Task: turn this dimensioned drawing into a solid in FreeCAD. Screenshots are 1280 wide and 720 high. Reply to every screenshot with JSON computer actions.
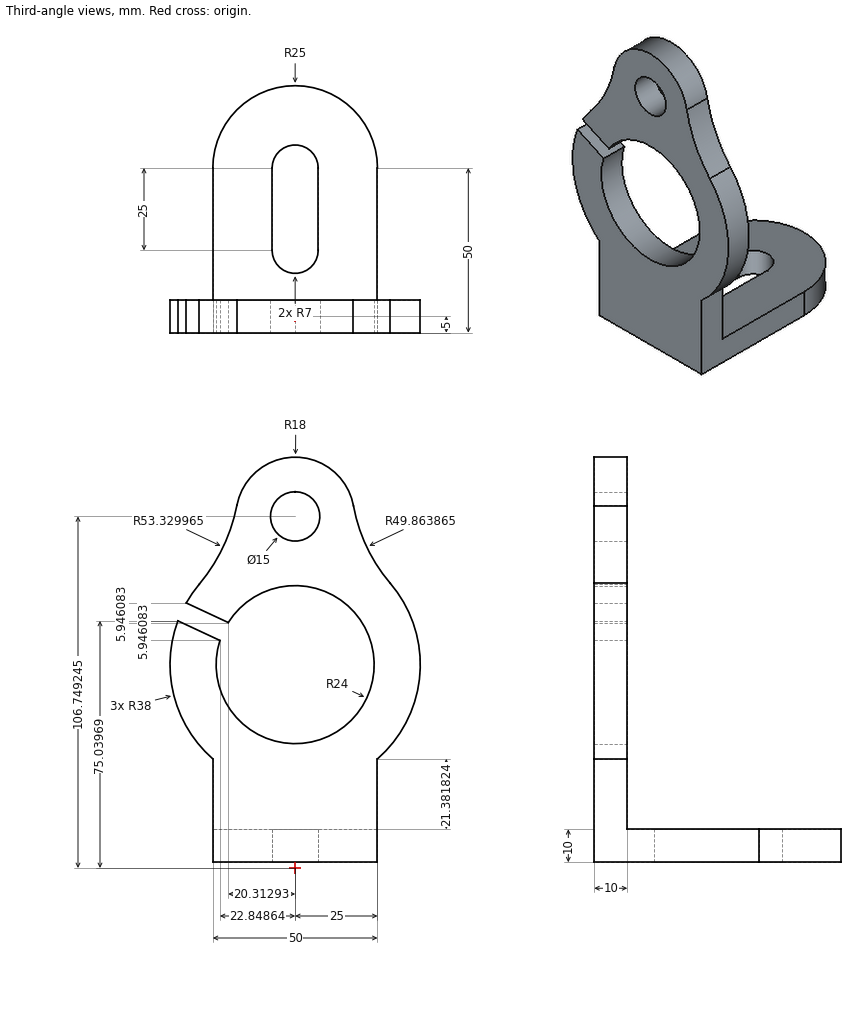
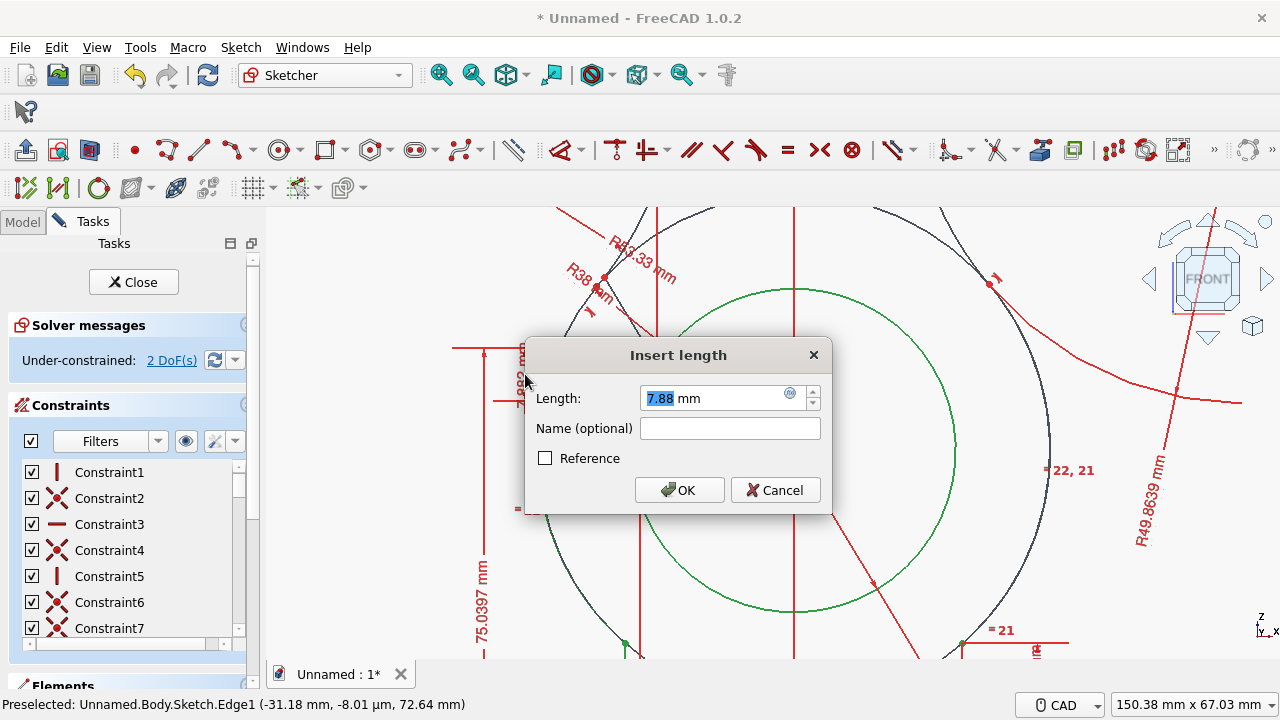
{"action": "type", "text": "5.946083"}
{"action": "key", "text": "Return"}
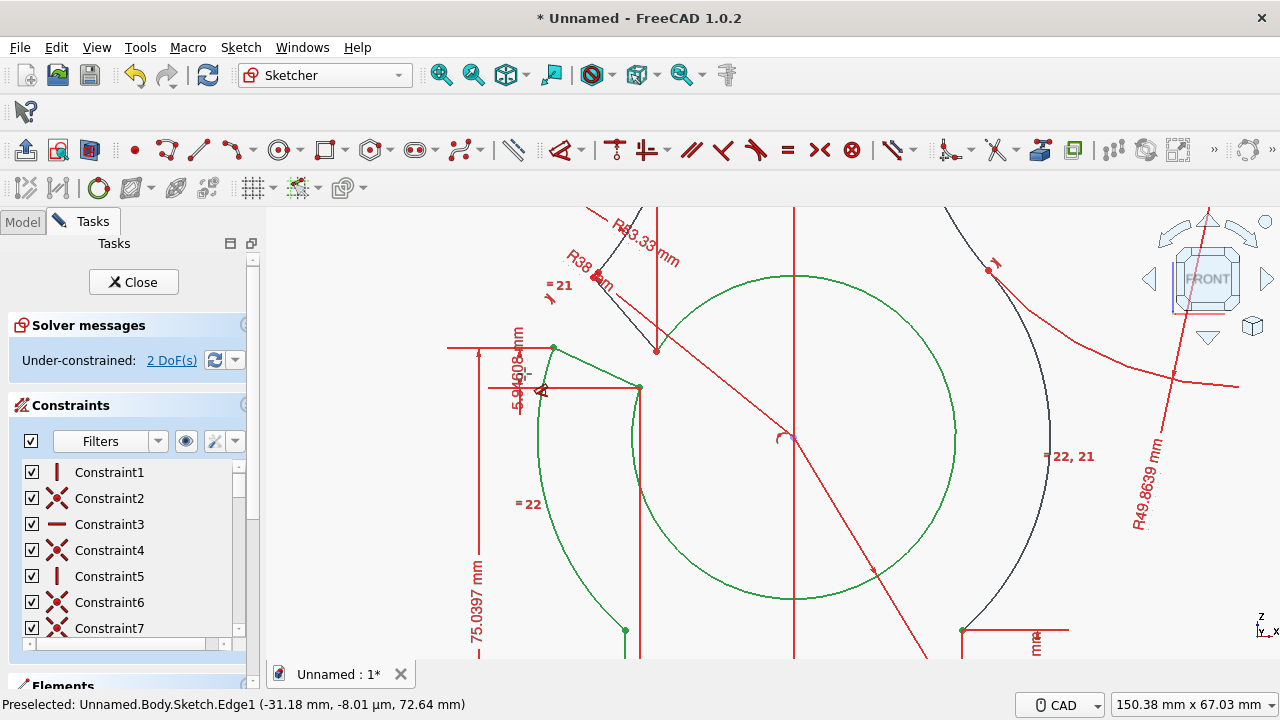
{"action": "left_click", "coordinate": [638, 329]}
{"action": "left_click", "coordinate": [560, 314]}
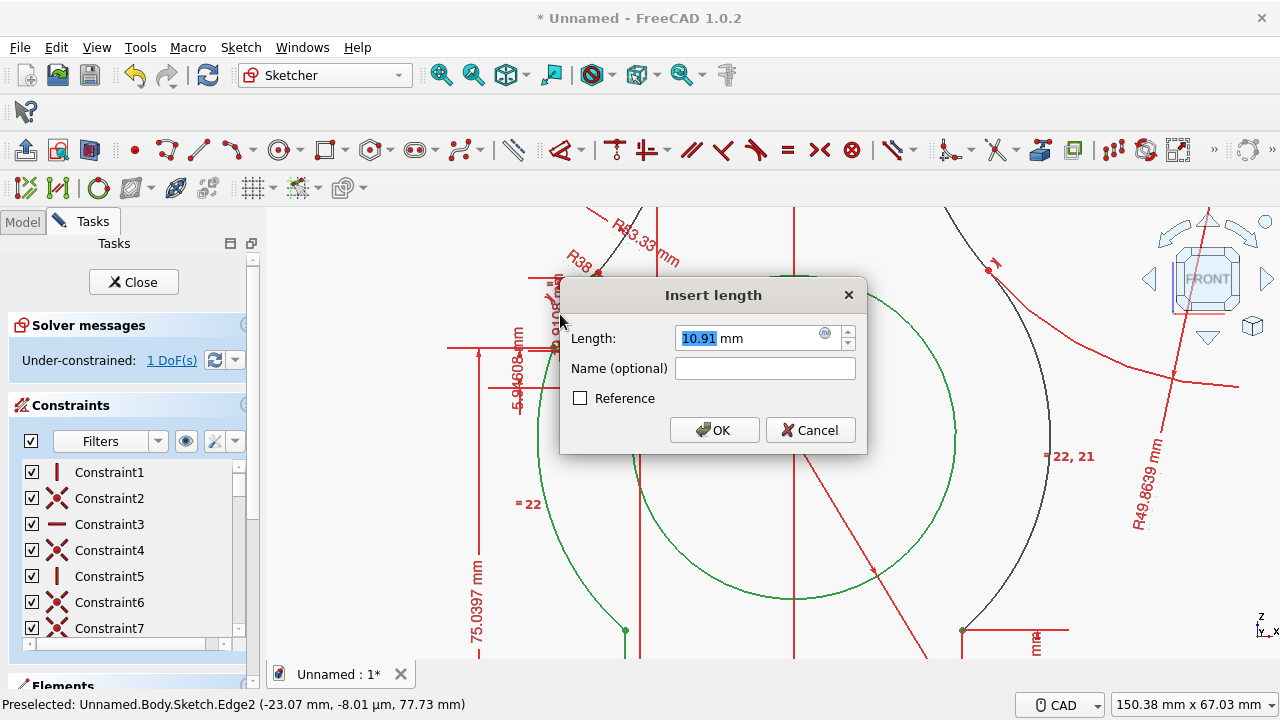
{"action": "type", "text": "5.946083"}
{"action": "key", "text": "Return"}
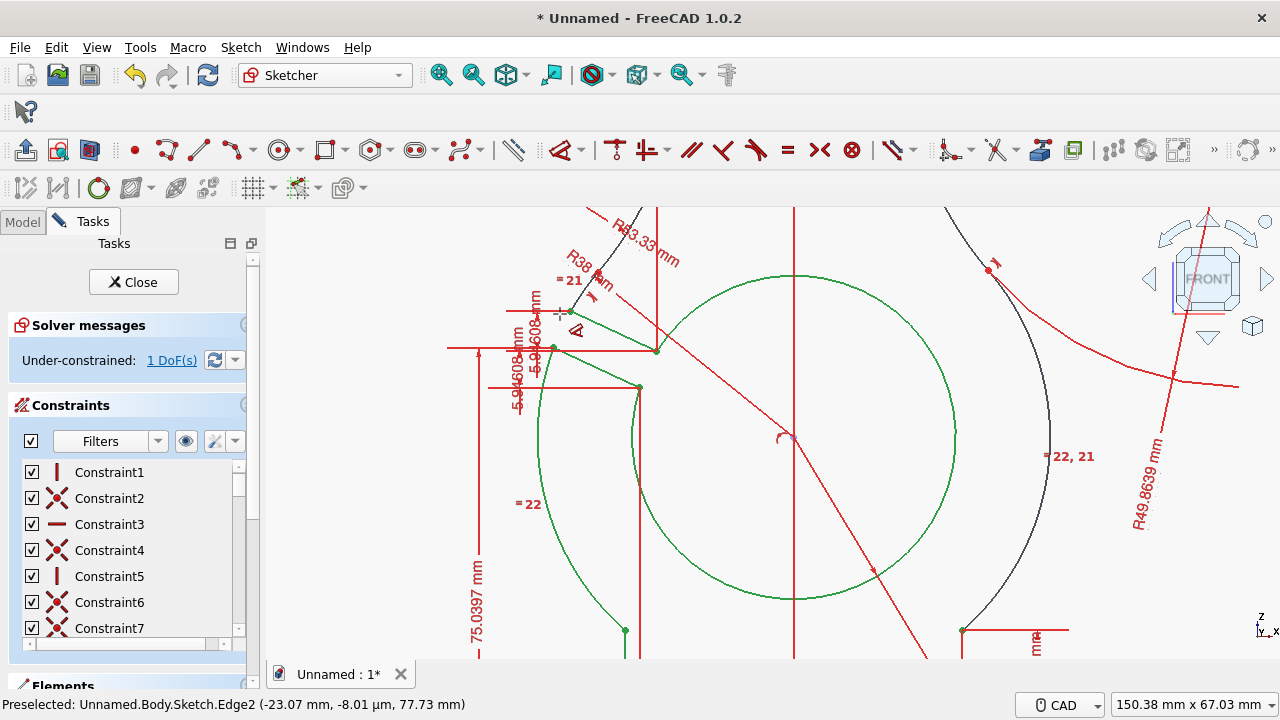
{"action": "scroll", "coordinate": [664, 433], "scroll_direction": "down", "scroll_amount": 6}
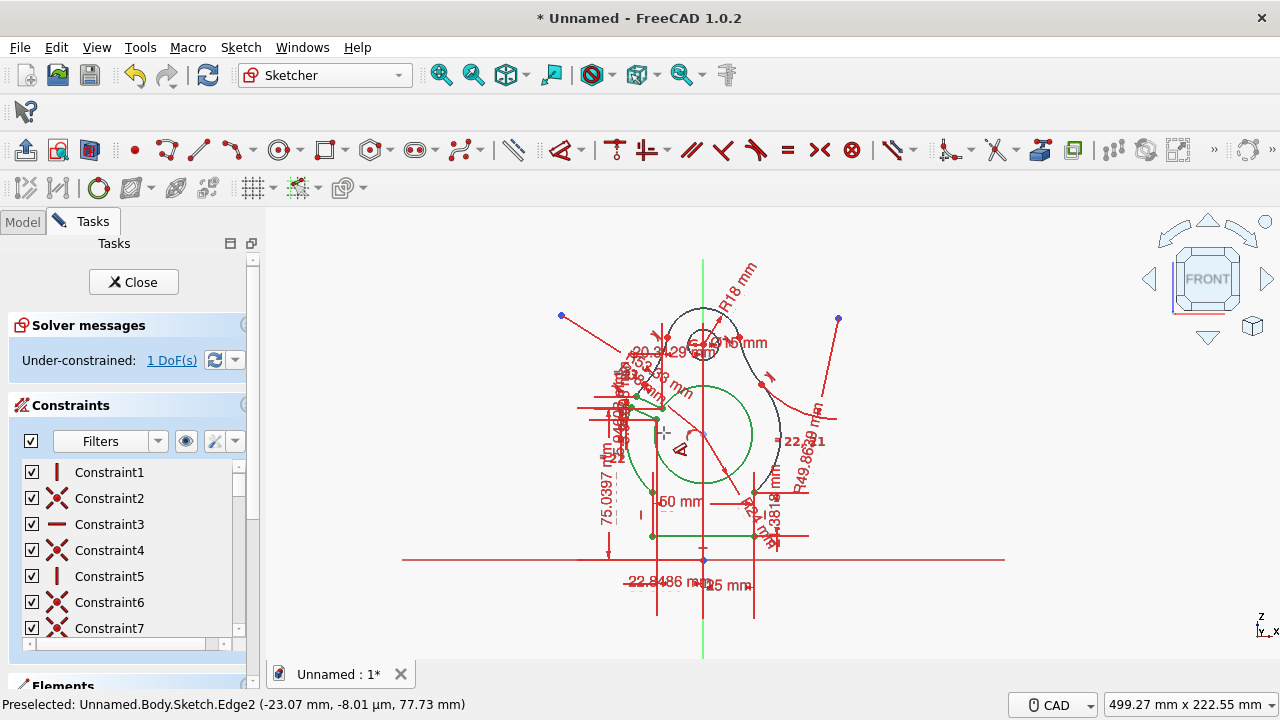
{"action": "left_click", "coordinate": [703, 345]}
{"action": "left_click", "coordinate": [737, 377]}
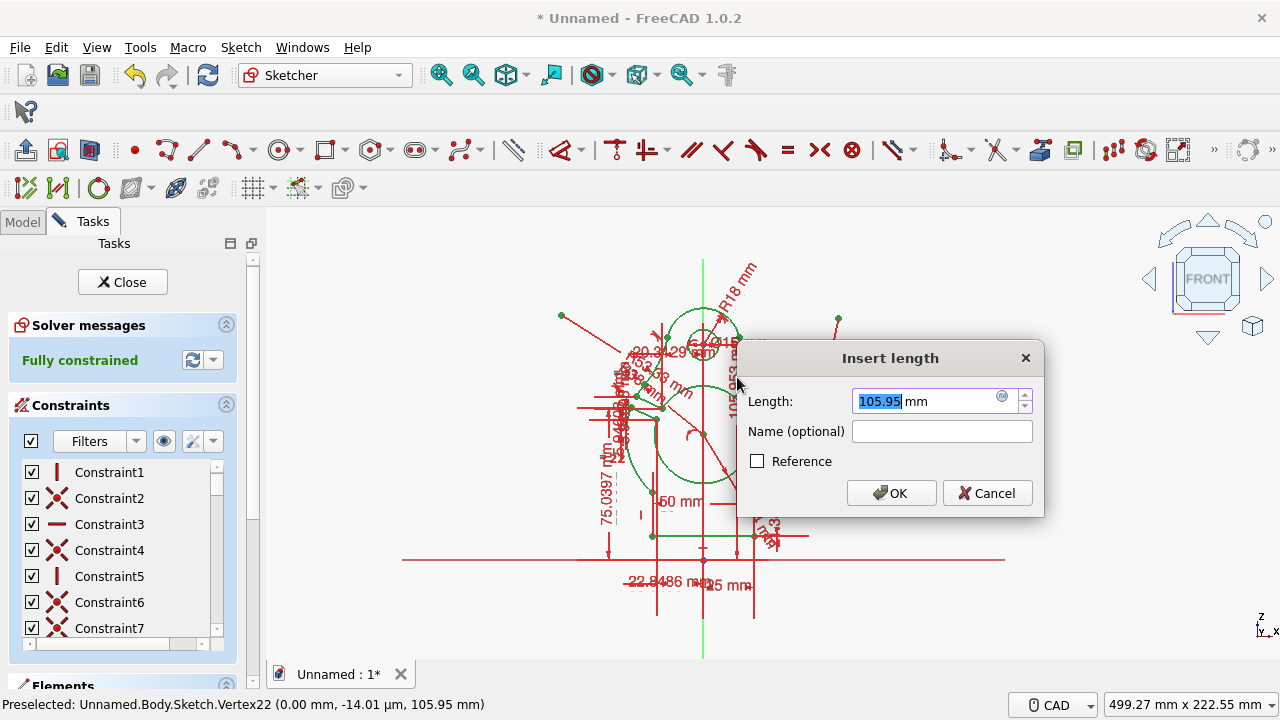
{"action": "type", "text": "106.749245"}
{"action": "key", "text": "Return"}
{"action": "key", "text": "Escape"}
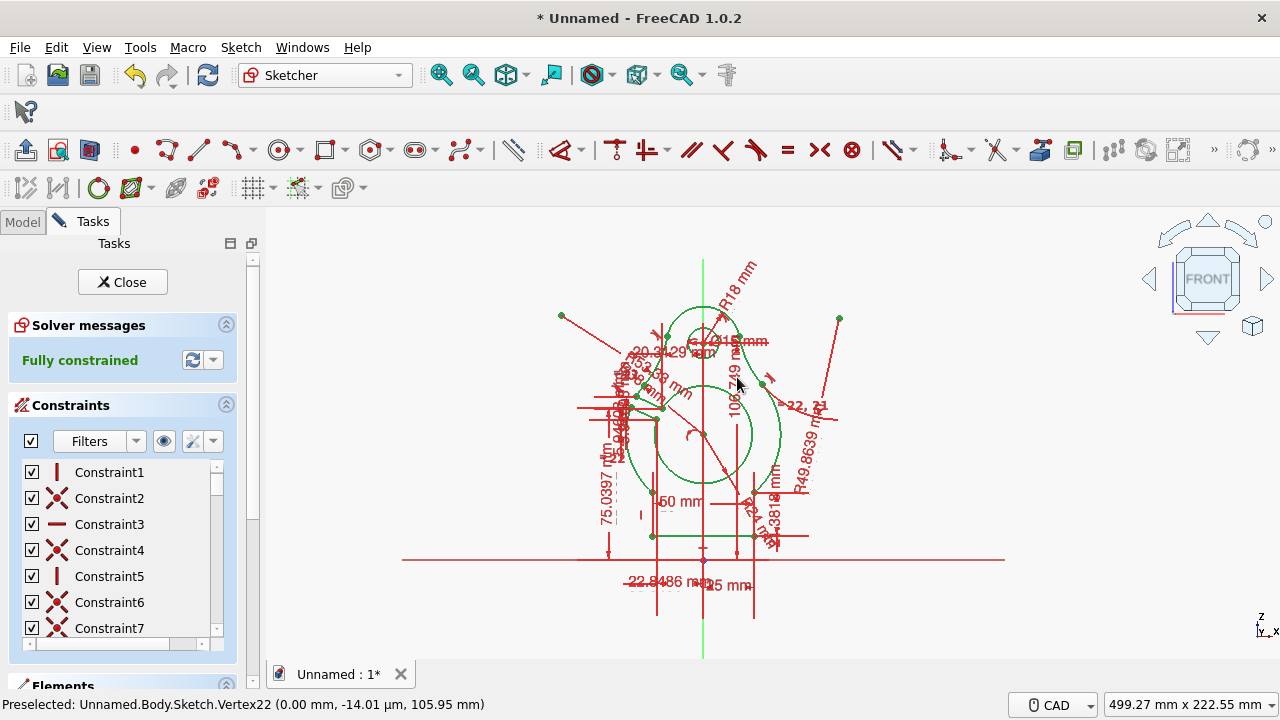
{"action": "left_click", "coordinate": [123, 282]}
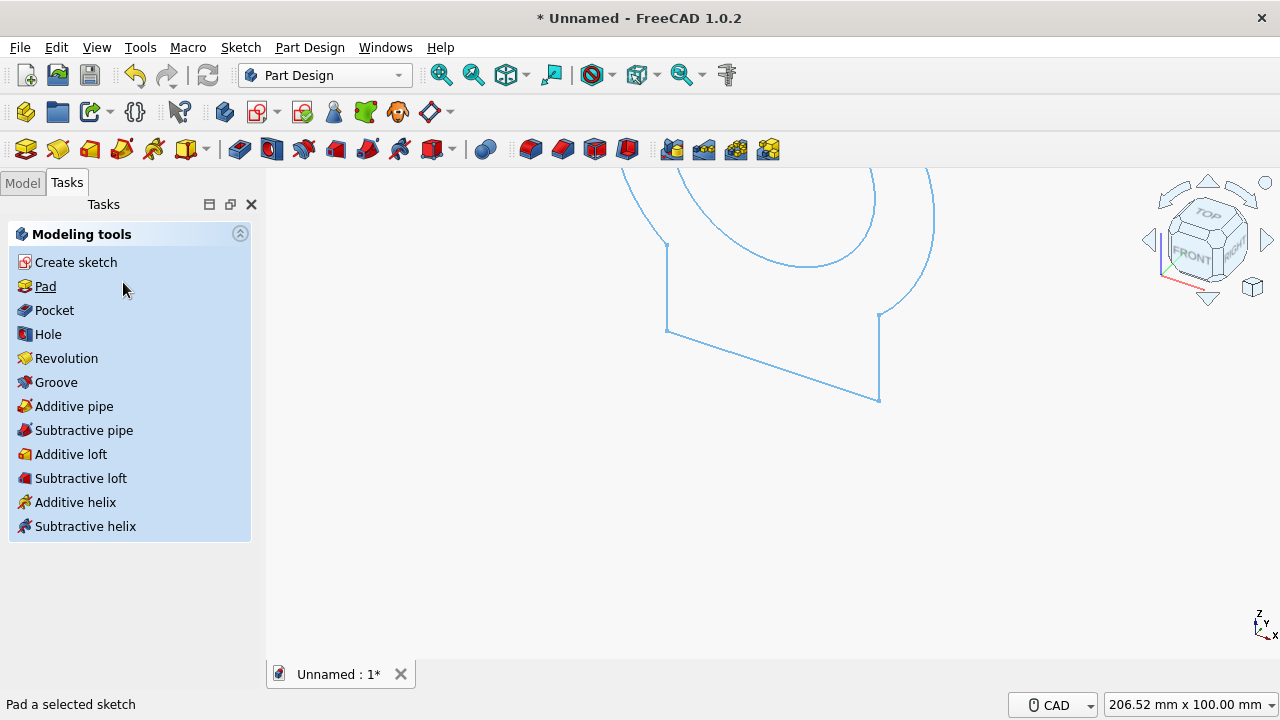
{"action": "left_click", "coordinate": [26, 150]}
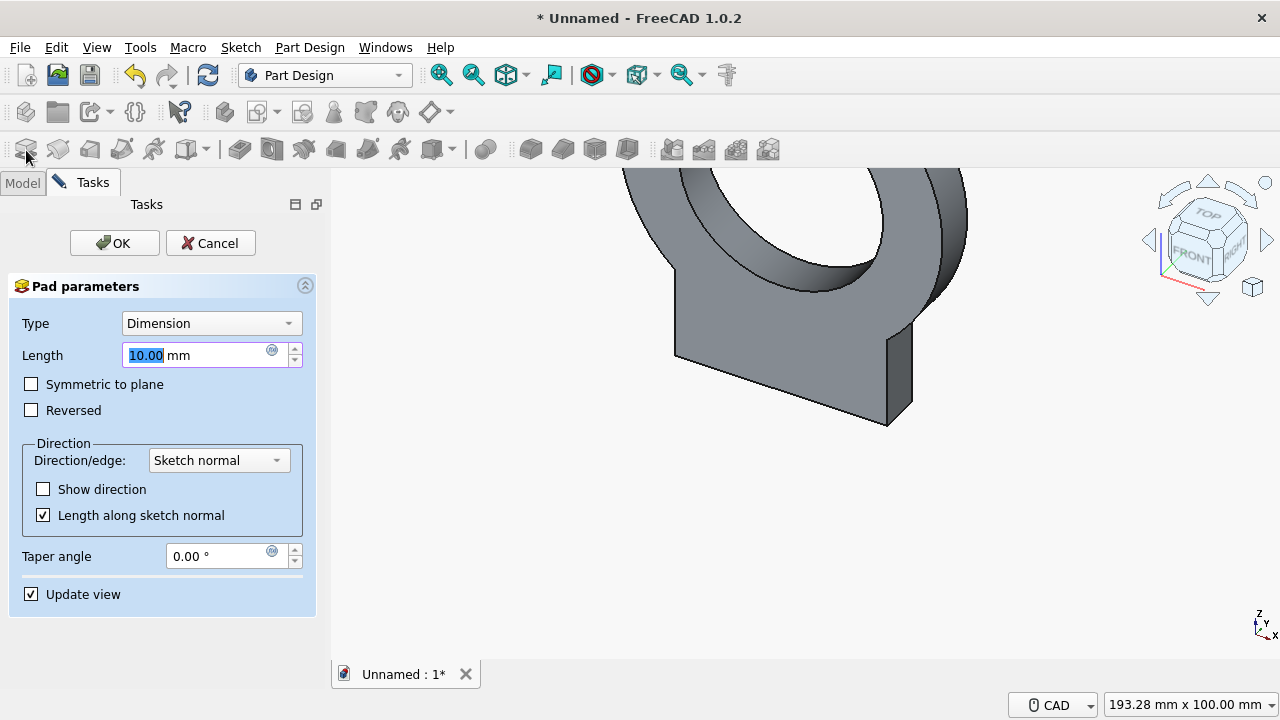
{"action": "type", "text": "10"}
{"action": "key", "text": "Tab"}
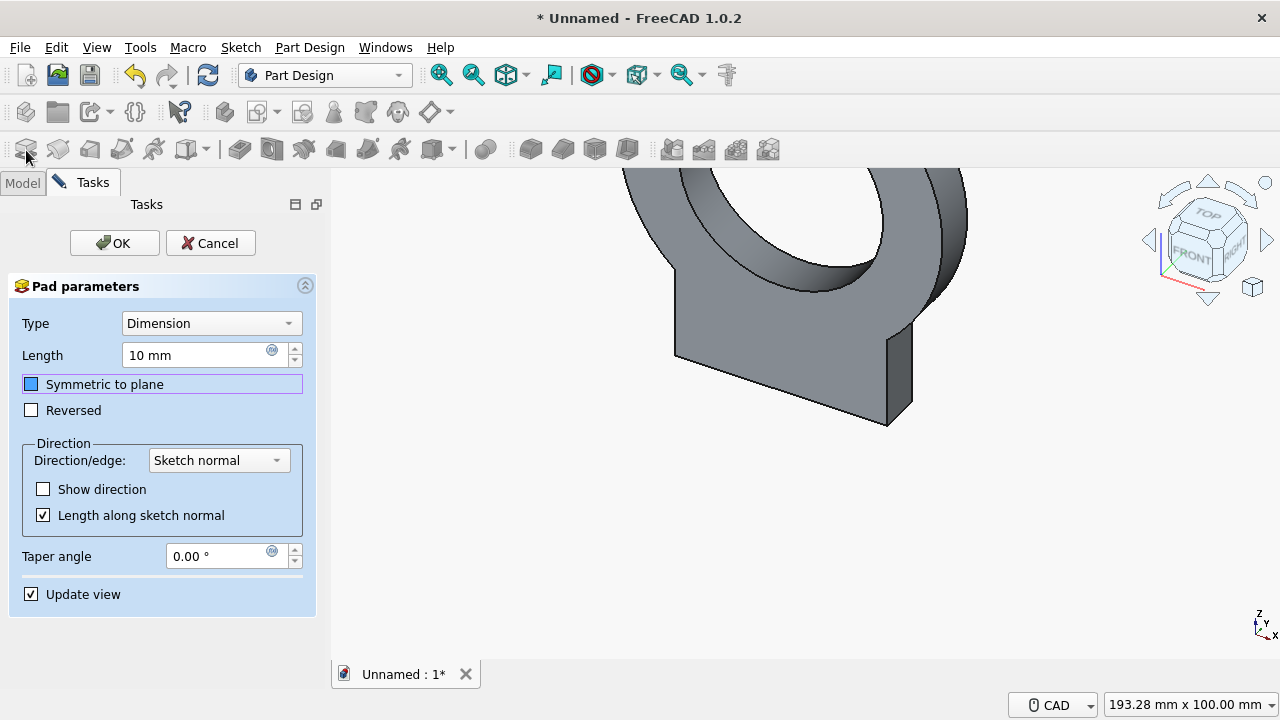
{"action": "left_click", "coordinate": [30, 384]}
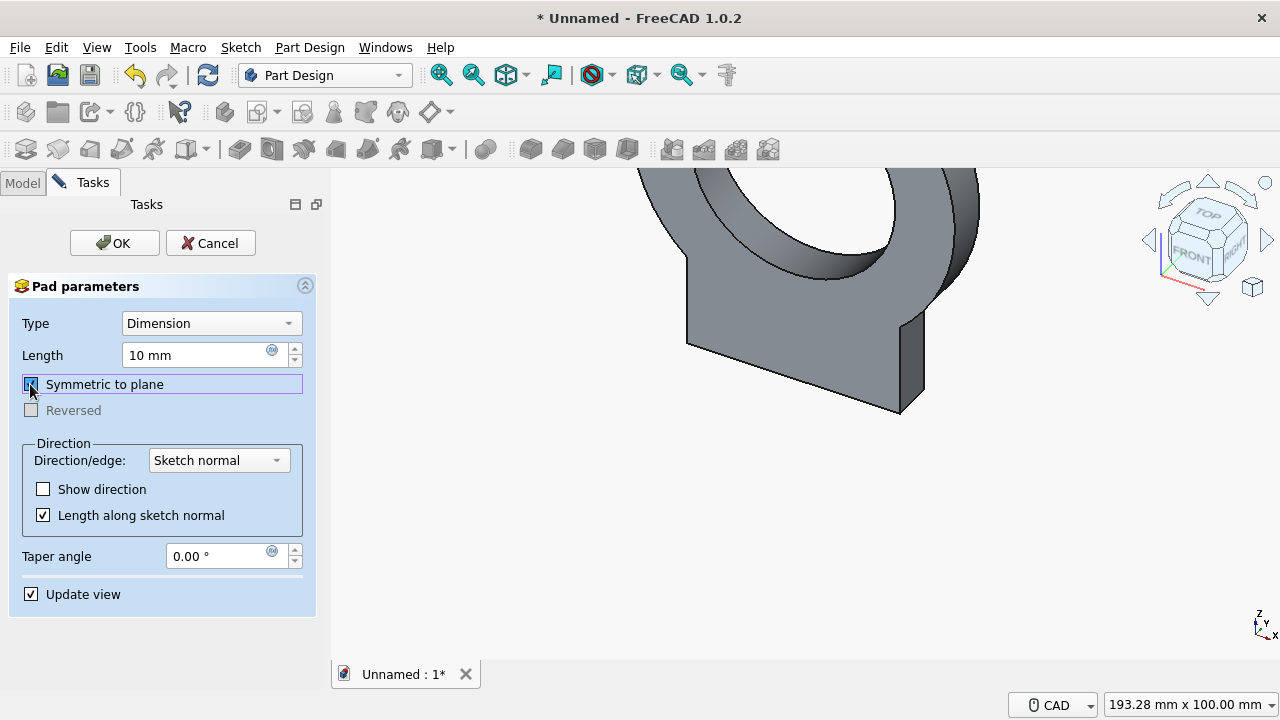
{"action": "left_click", "coordinate": [115, 243]}